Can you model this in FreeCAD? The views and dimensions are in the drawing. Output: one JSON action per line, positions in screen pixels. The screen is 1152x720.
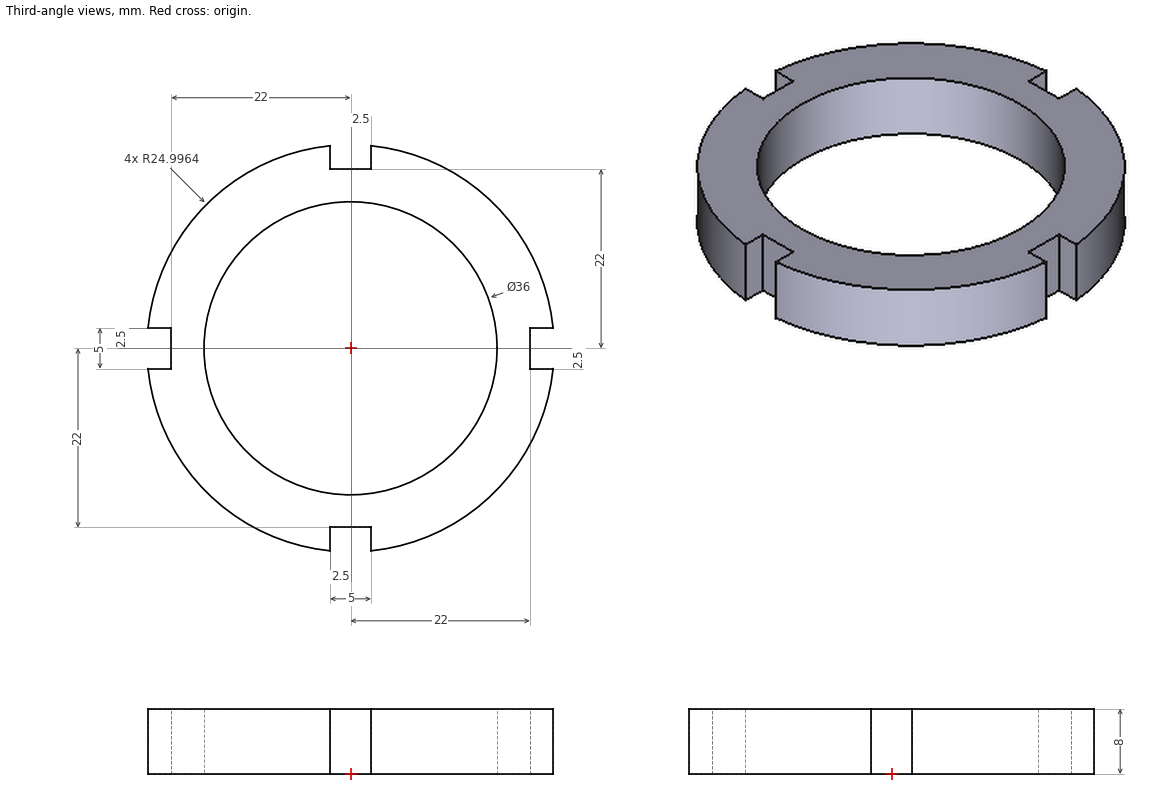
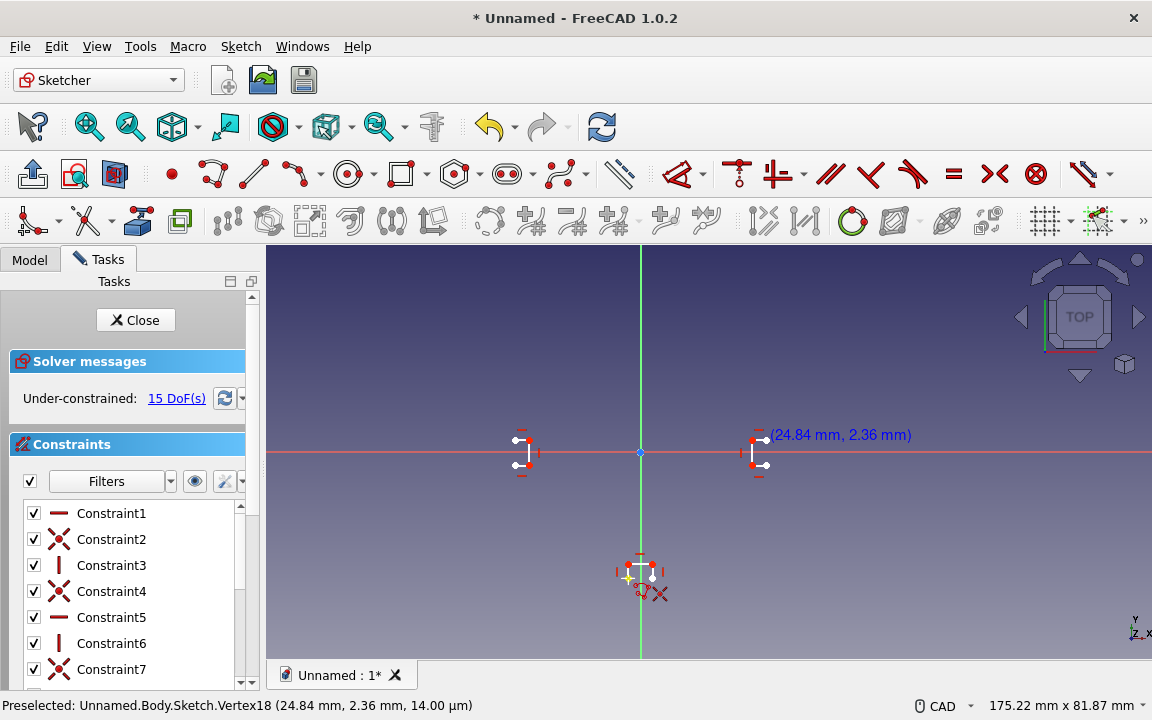
{"action": "scroll", "coordinate": [653, 326], "scroll_direction": "up", "scroll_amount": 2}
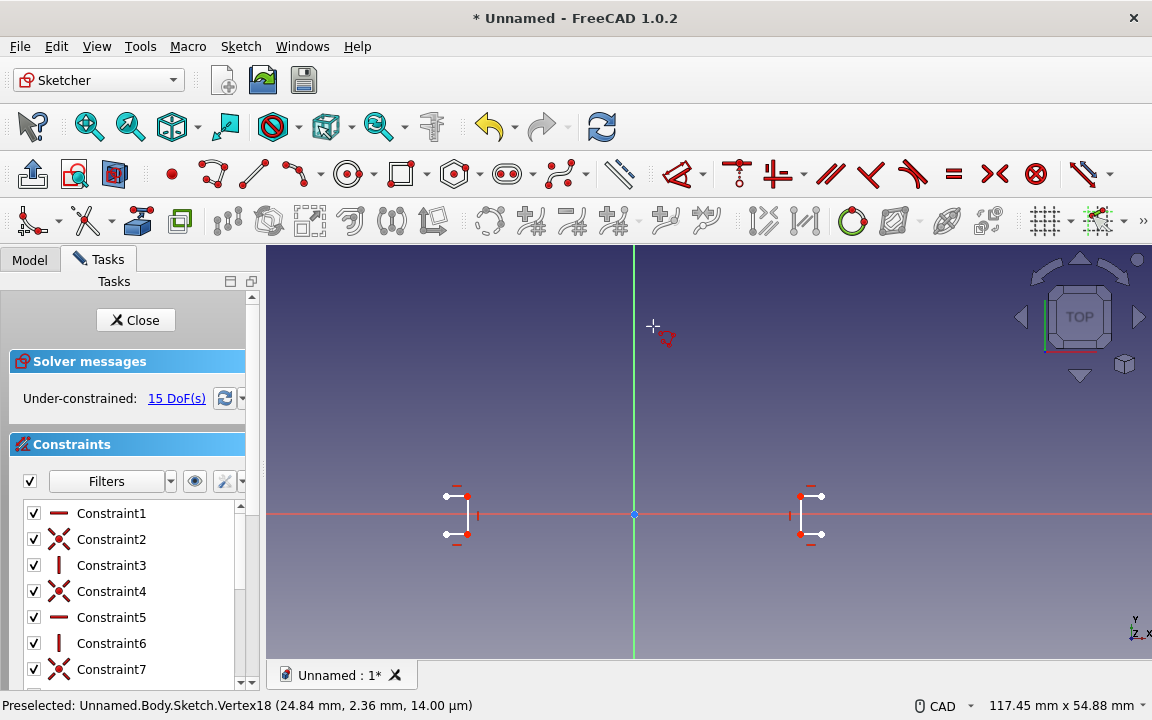
{"action": "left_click", "coordinate": [653, 326]}
{"action": "left_click", "coordinate": [653, 348]}
{"action": "left_click", "coordinate": [615, 348]}
{"action": "left_click", "coordinate": [615, 326]}
{"action": "right_click", "coordinate": [615, 326]}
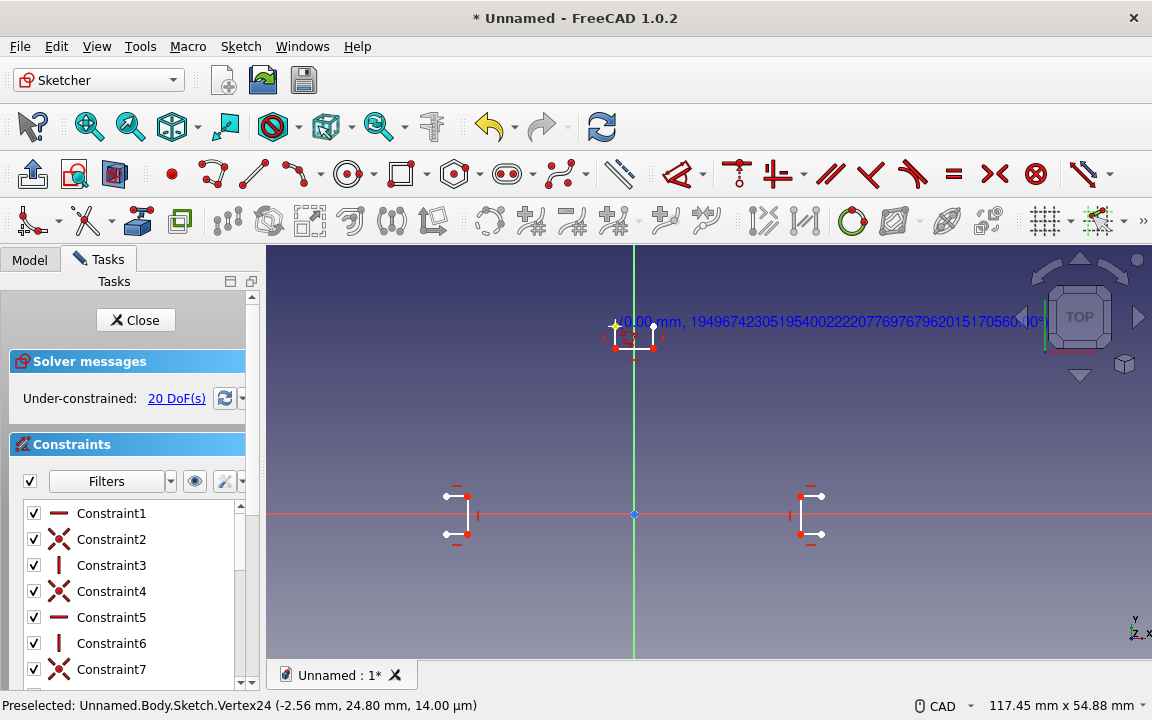
{"action": "key", "text": "g 3 a"}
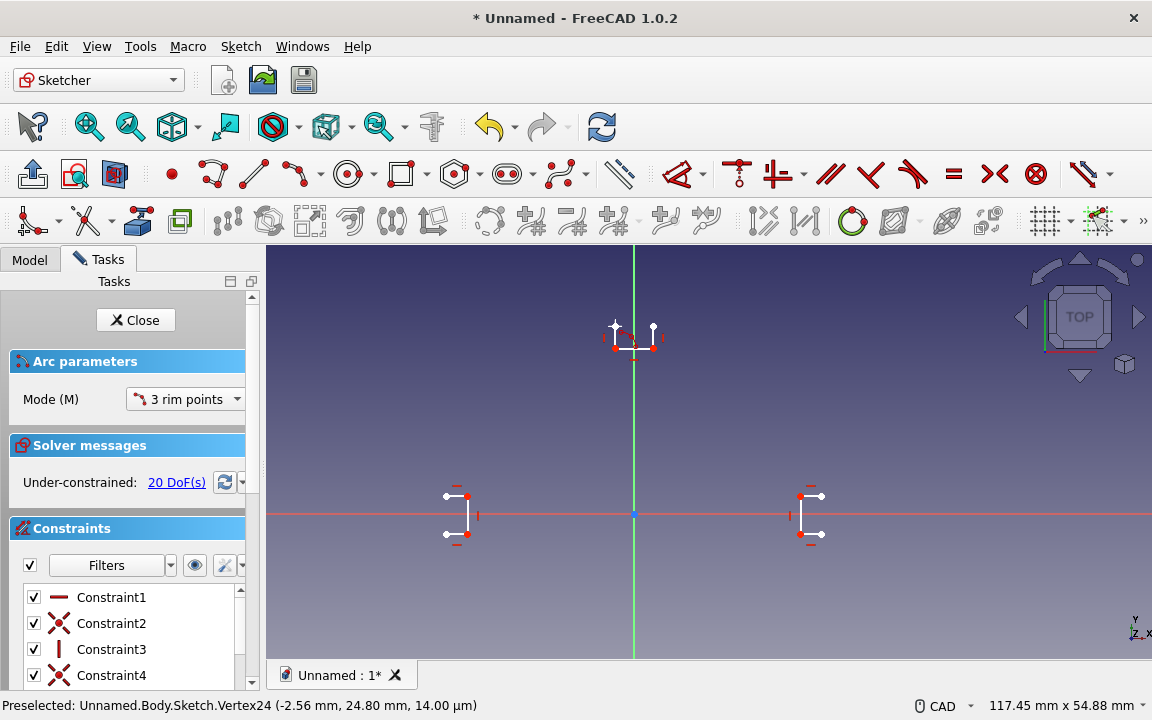
{"action": "scroll", "coordinate": [447, 533], "scroll_direction": "up", "scroll_amount": 2}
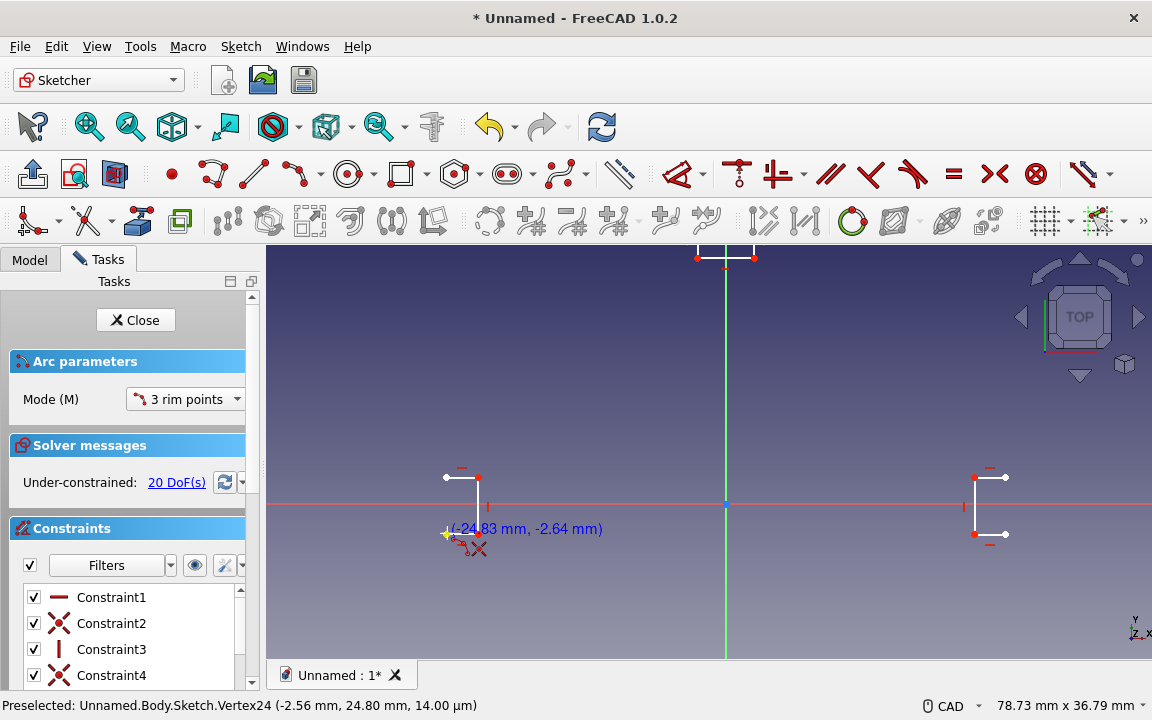
{"action": "left_click", "coordinate": [447, 534]}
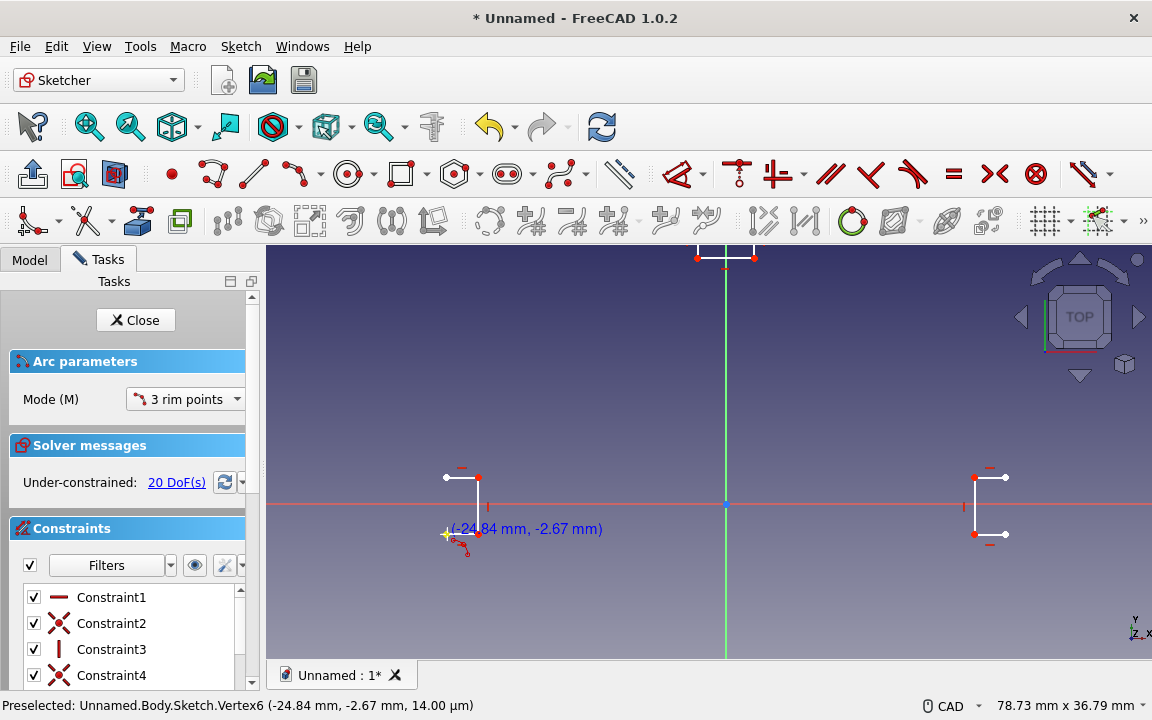
{"action": "scroll", "coordinate": [570, 409], "scroll_direction": "down", "scroll_amount": 4}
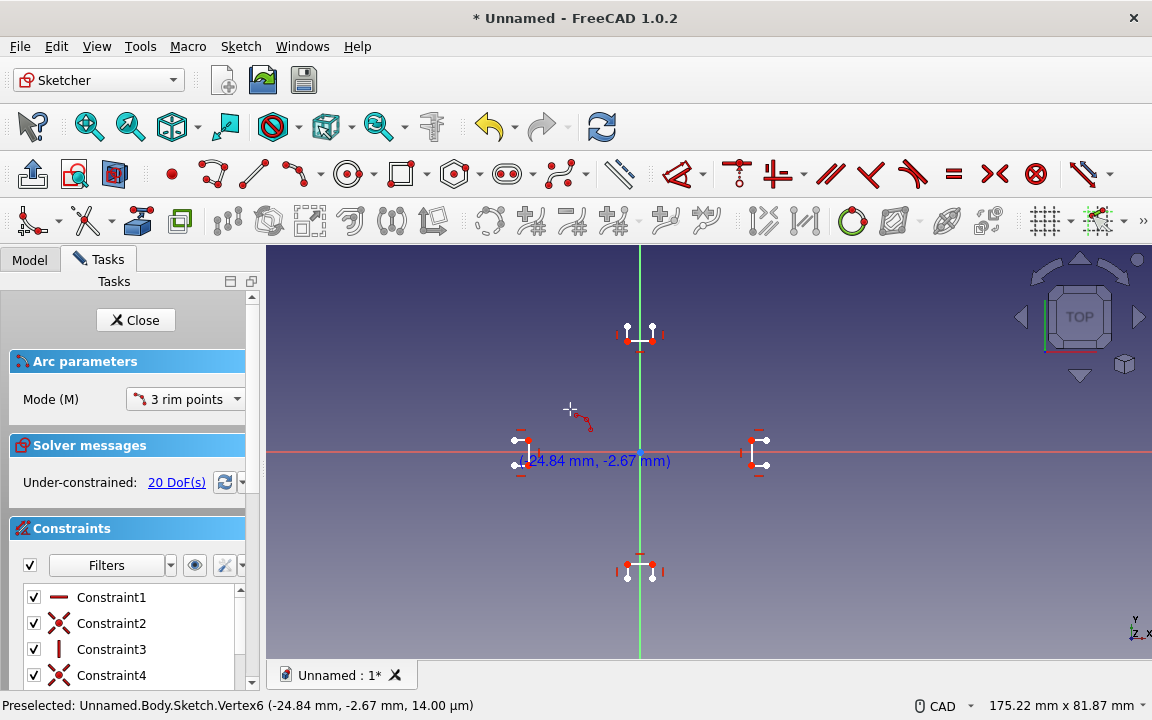
{"action": "scroll", "coordinate": [628, 578], "scroll_direction": "up", "scroll_amount": 4}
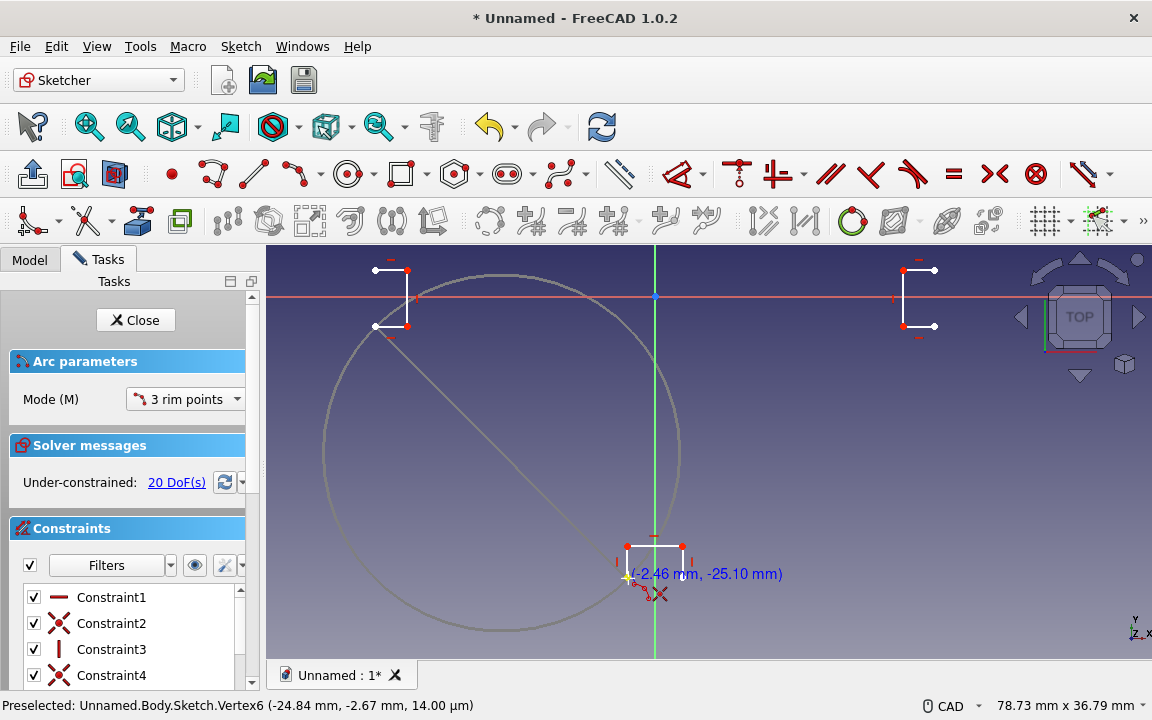
{"action": "left_click", "coordinate": [627, 578]}
{"action": "left_click", "coordinate": [456, 496]}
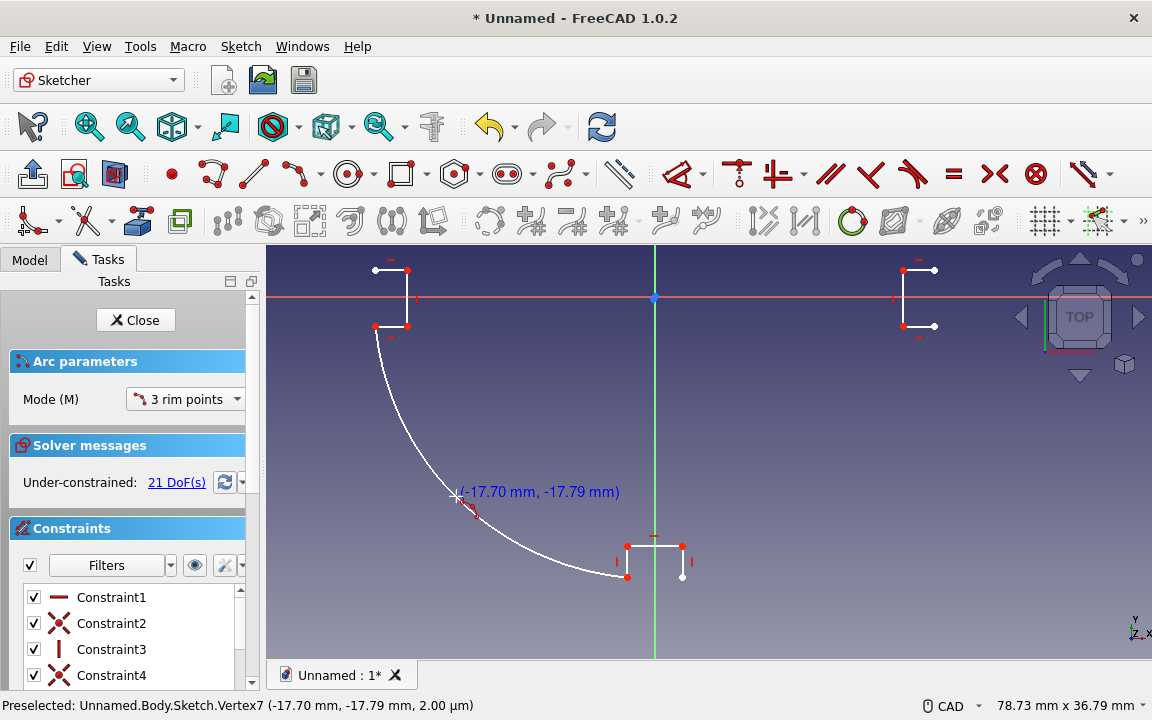
{"action": "left_click", "coordinate": [683, 578]}
{"action": "left_click", "coordinate": [935, 327]}
{"action": "left_click", "coordinate": [854, 496]}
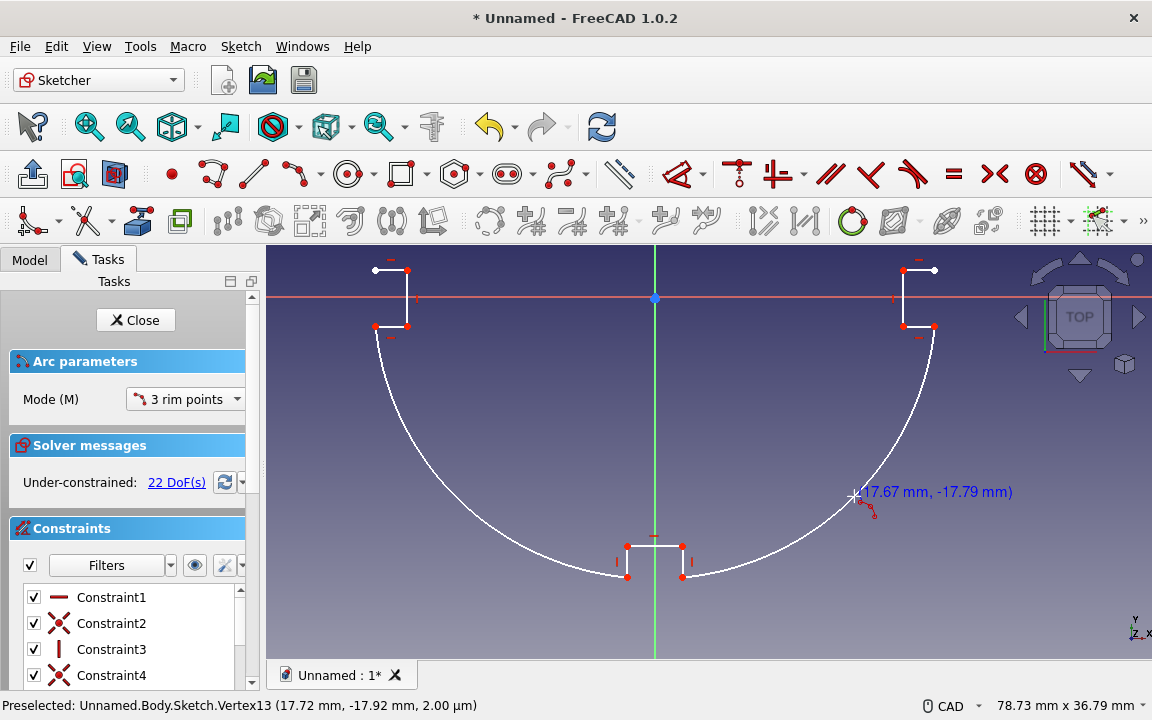
{"action": "scroll", "coordinate": [629, 579], "scroll_direction": "down", "scroll_amount": 4}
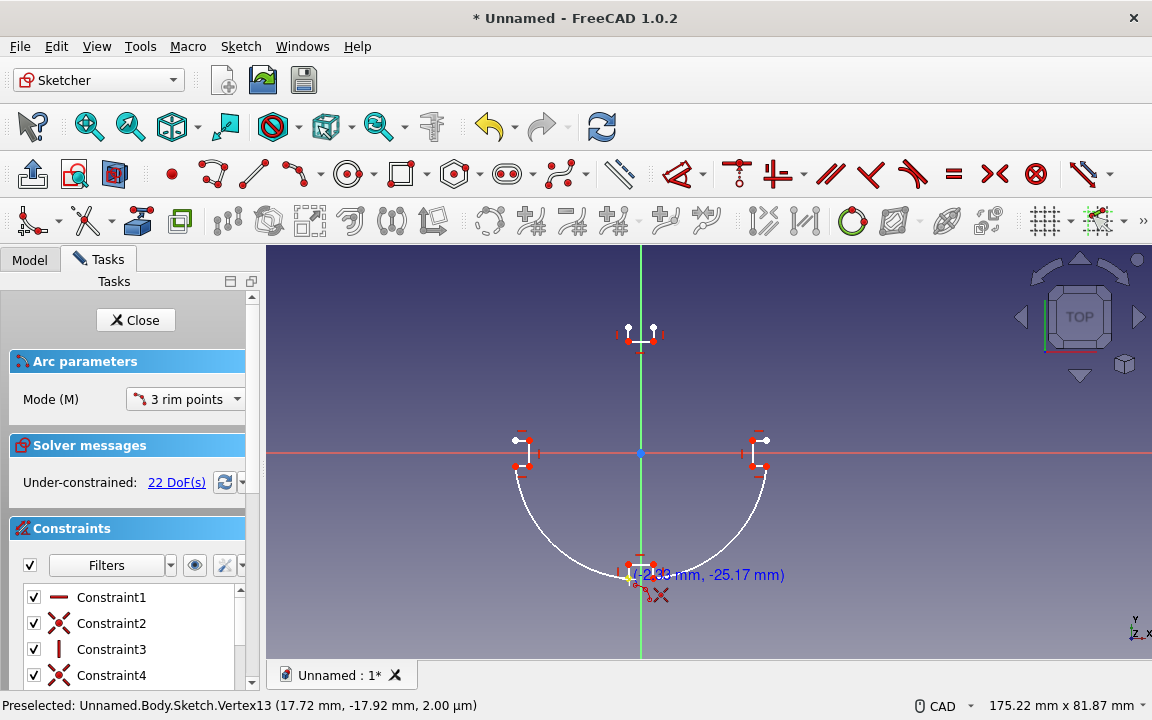
{"action": "scroll", "coordinate": [767, 440], "scroll_direction": "up", "scroll_amount": 4}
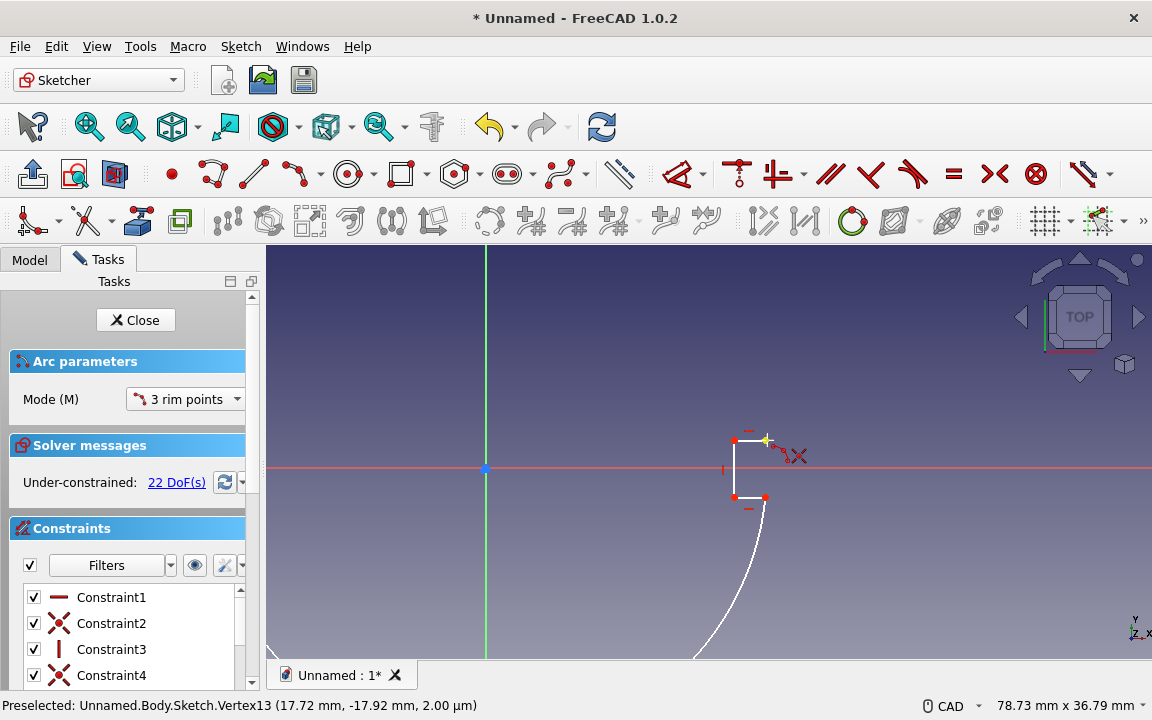
{"action": "left_click", "coordinate": [765, 441]}